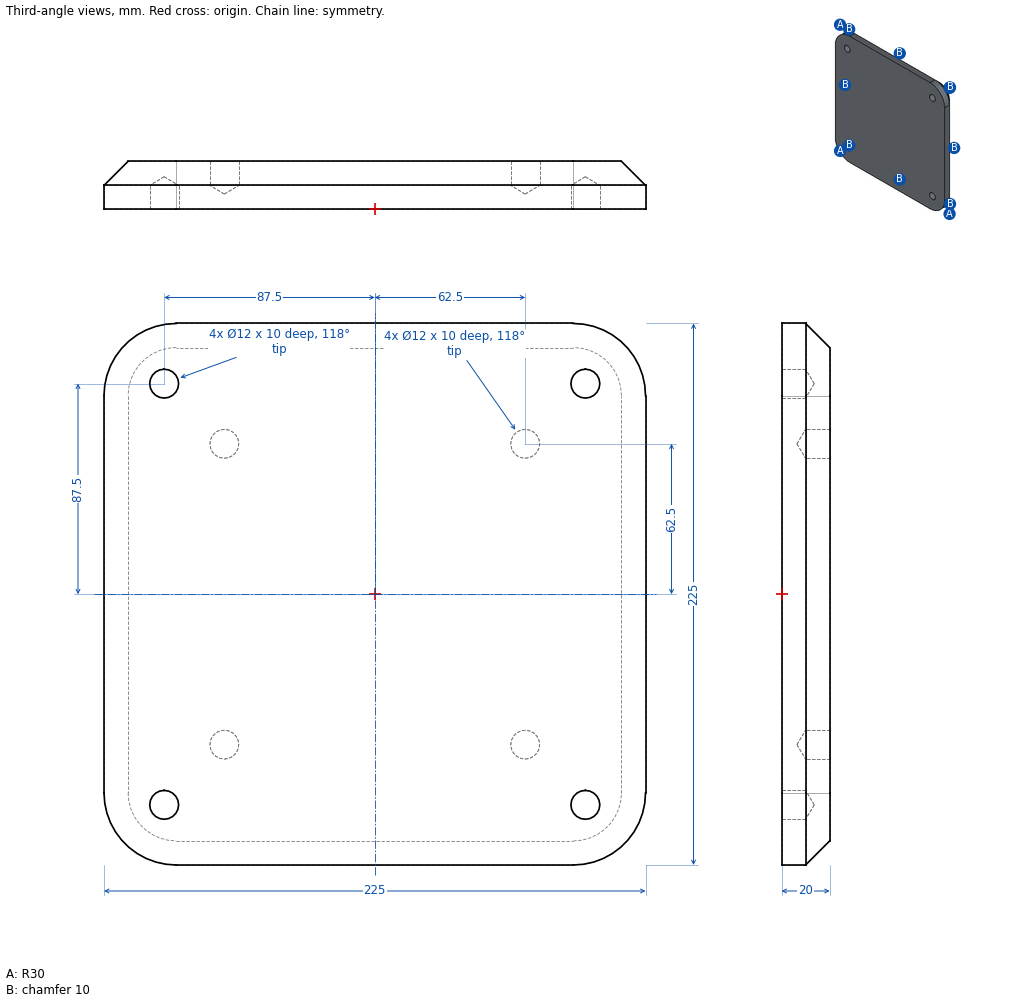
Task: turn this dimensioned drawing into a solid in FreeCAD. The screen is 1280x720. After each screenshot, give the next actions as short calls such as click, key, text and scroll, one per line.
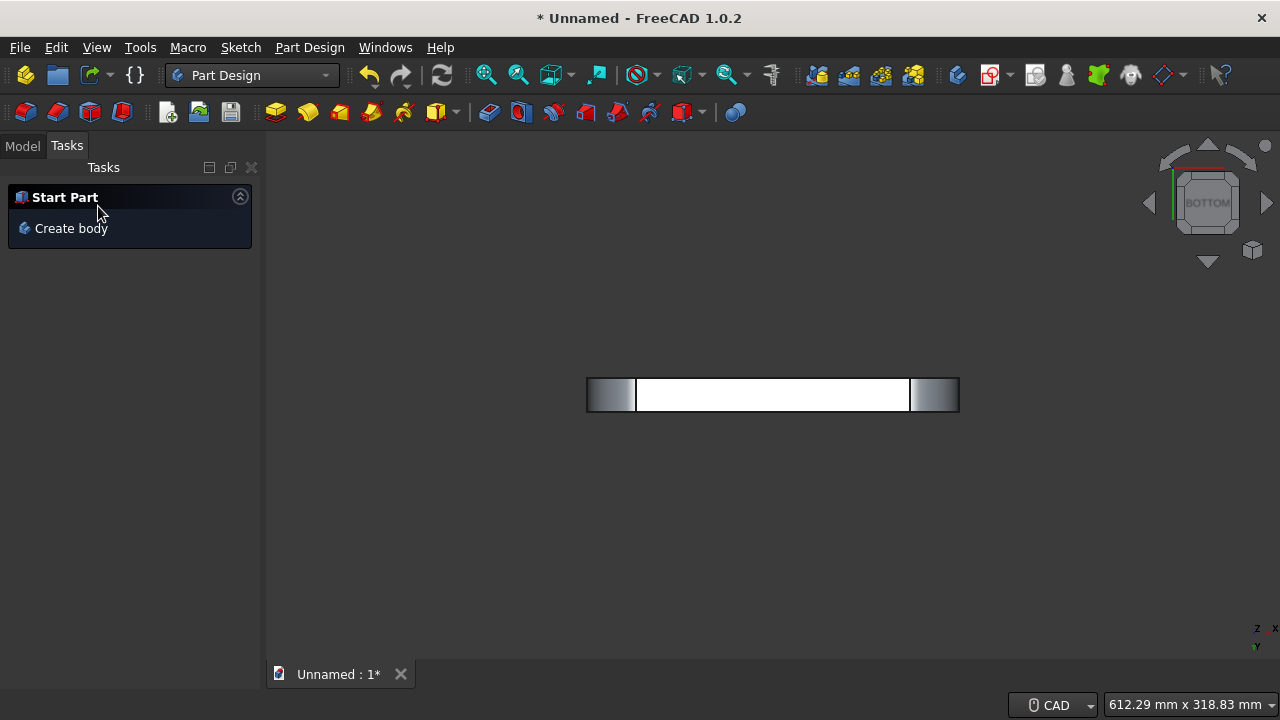
click(488, 76)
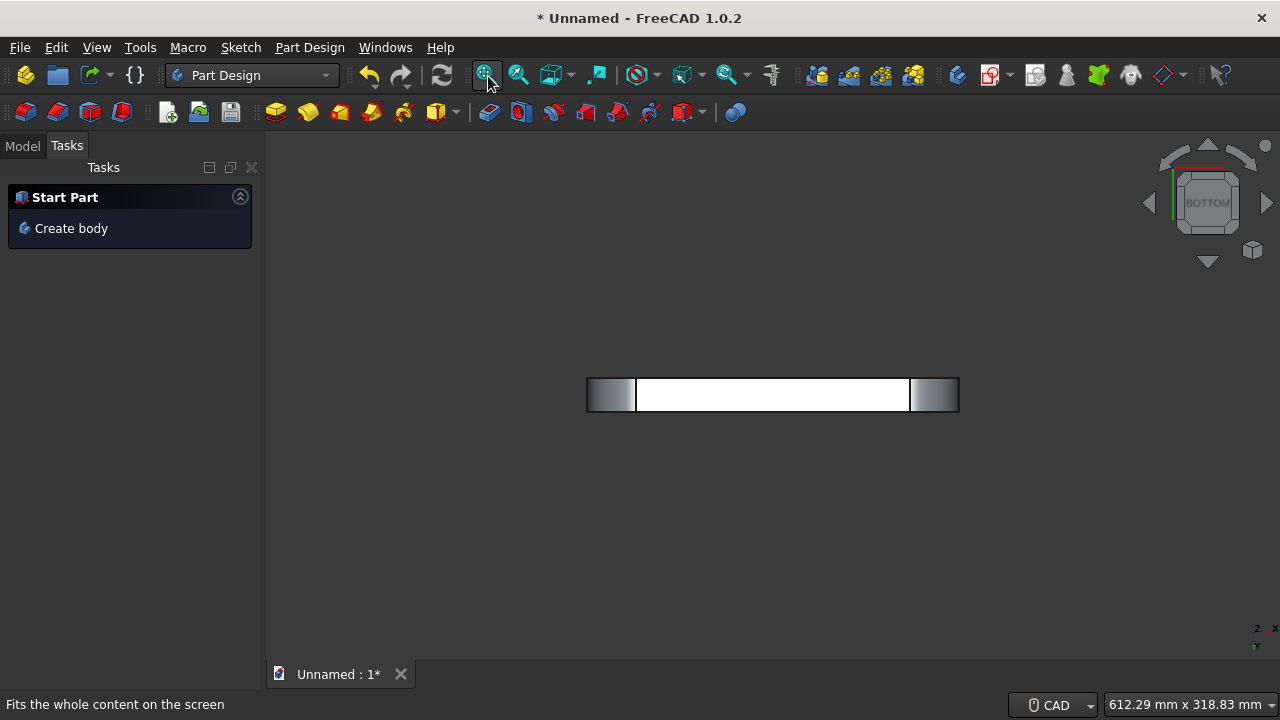
key(0)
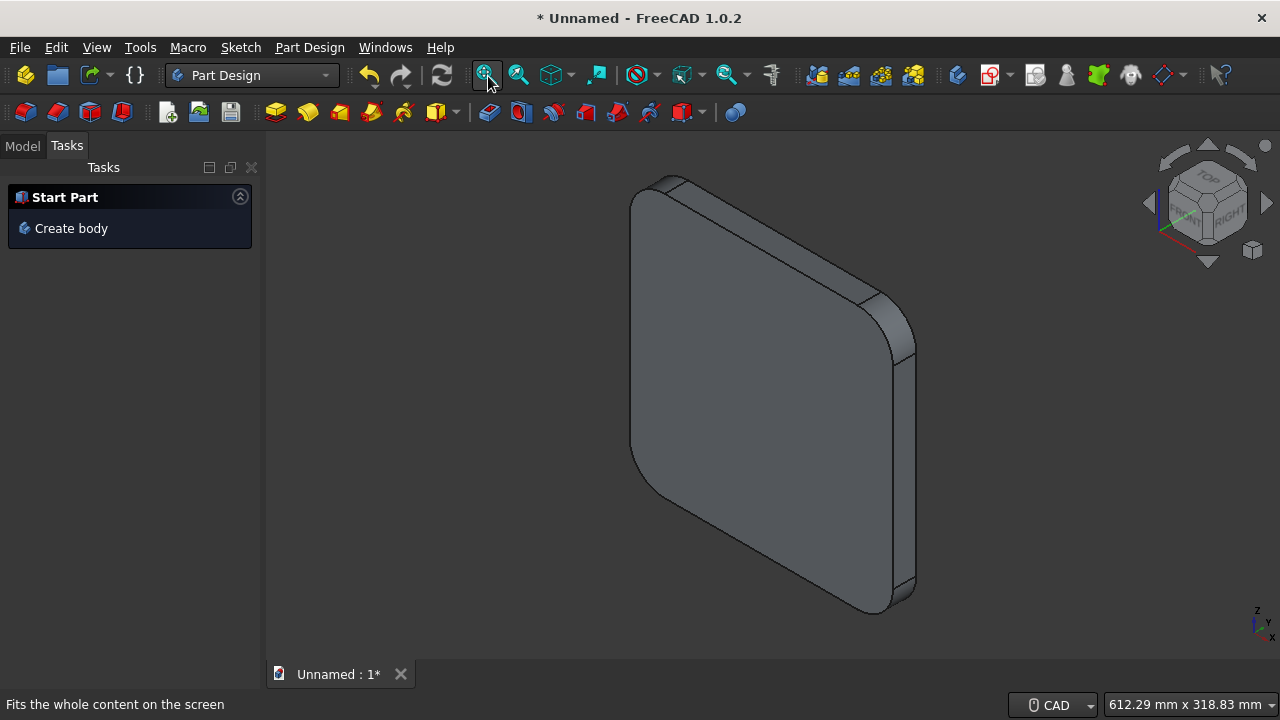
key(2)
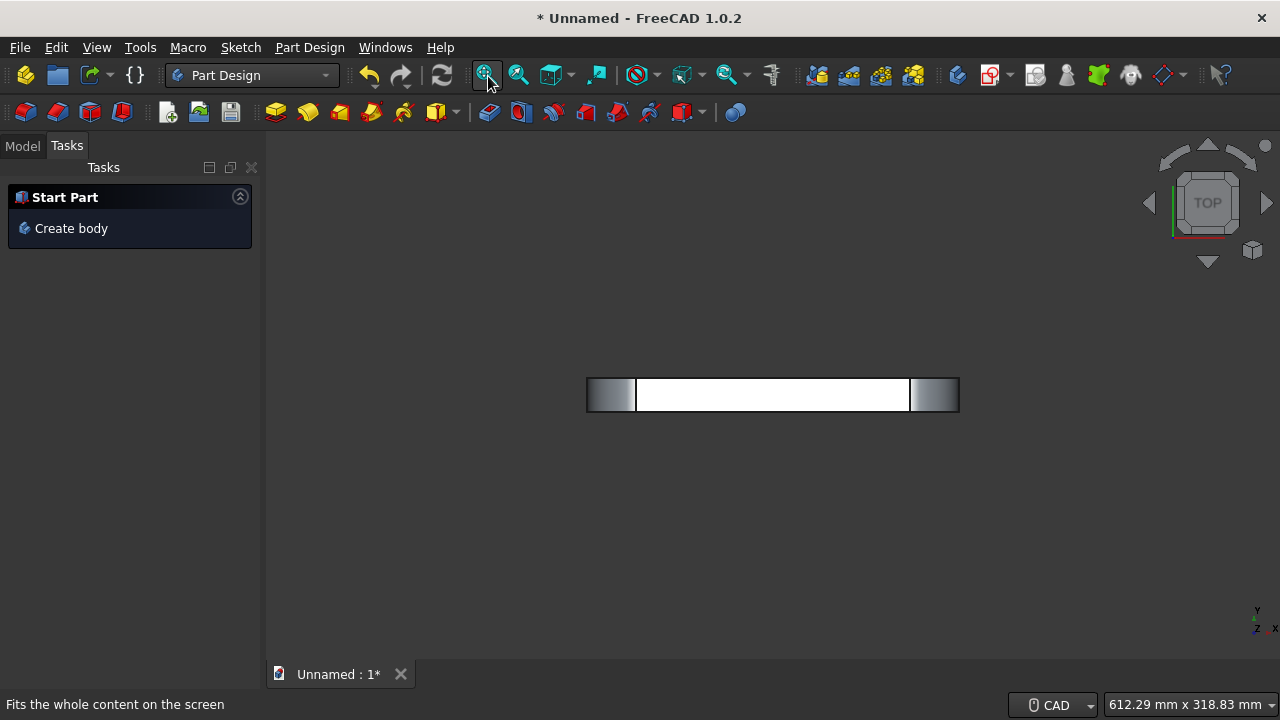
click(488, 76)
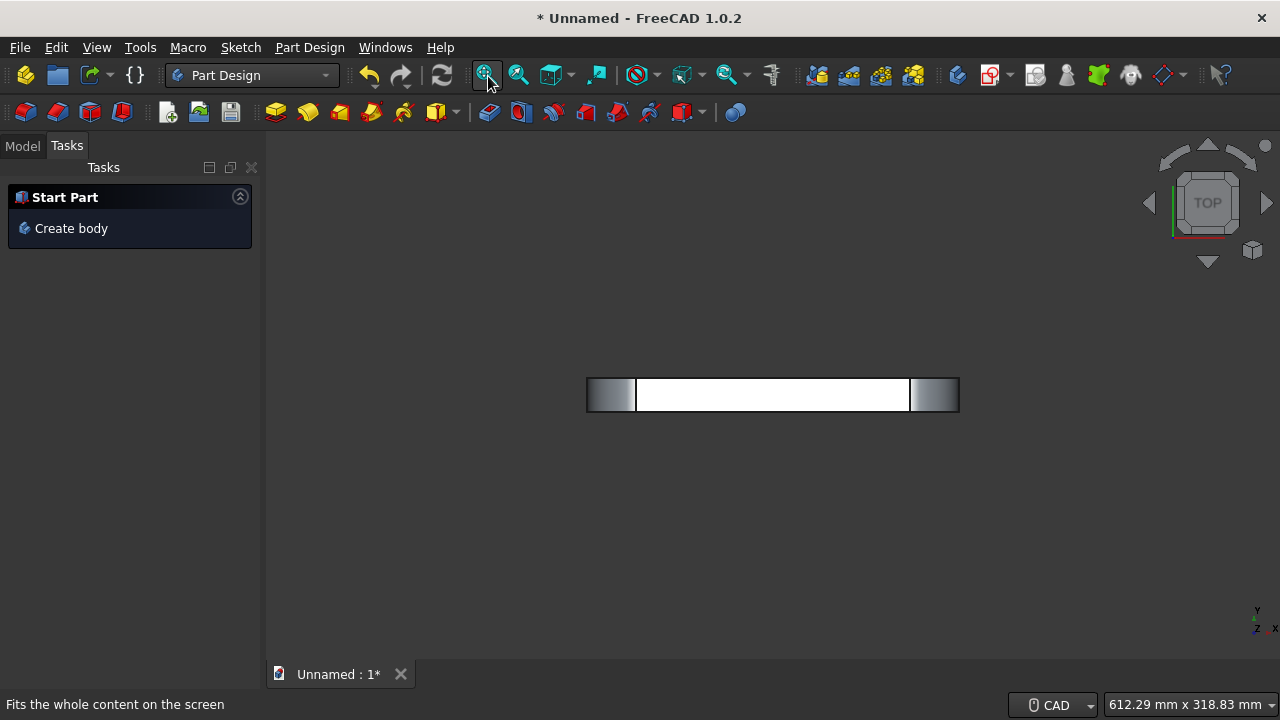
key(1)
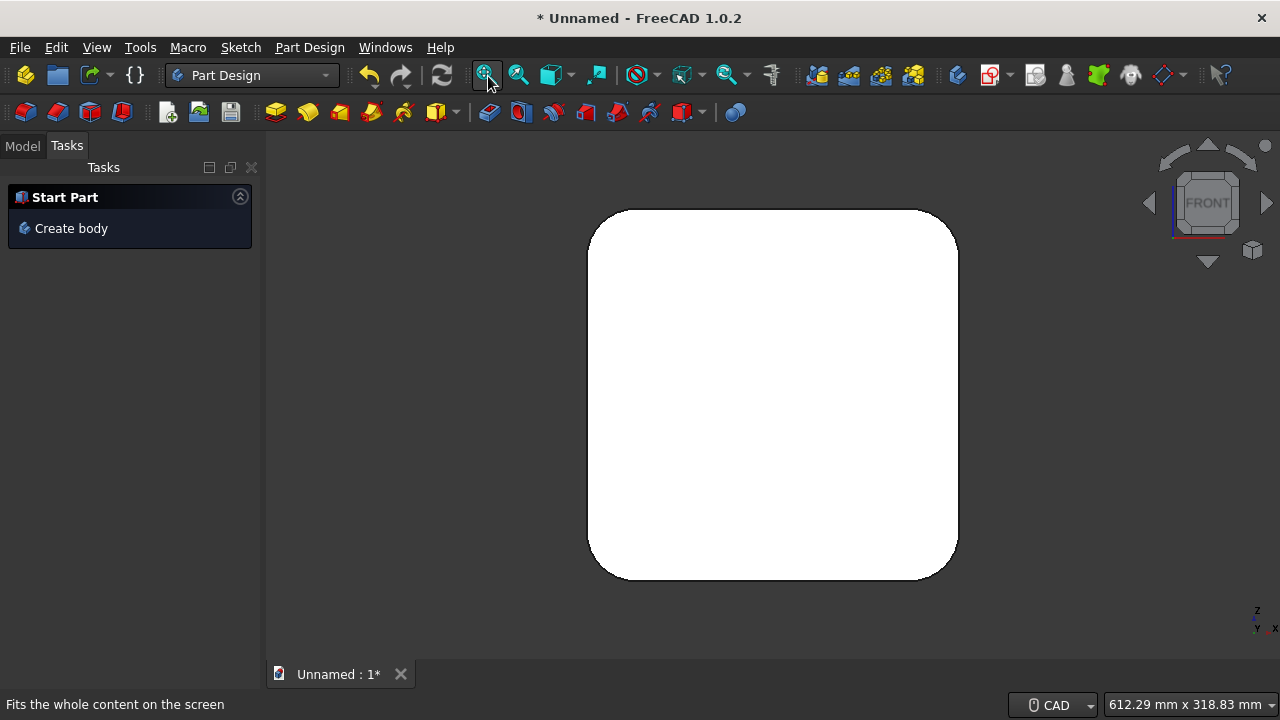
key(3)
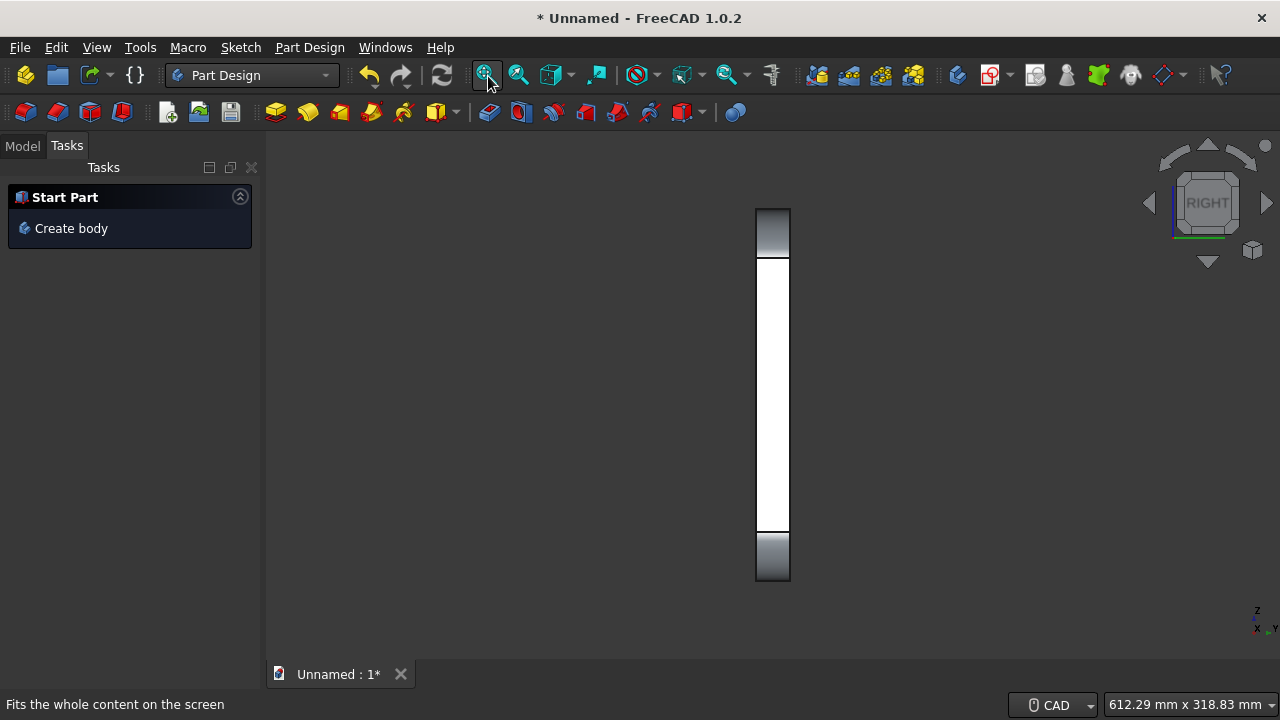
key(5)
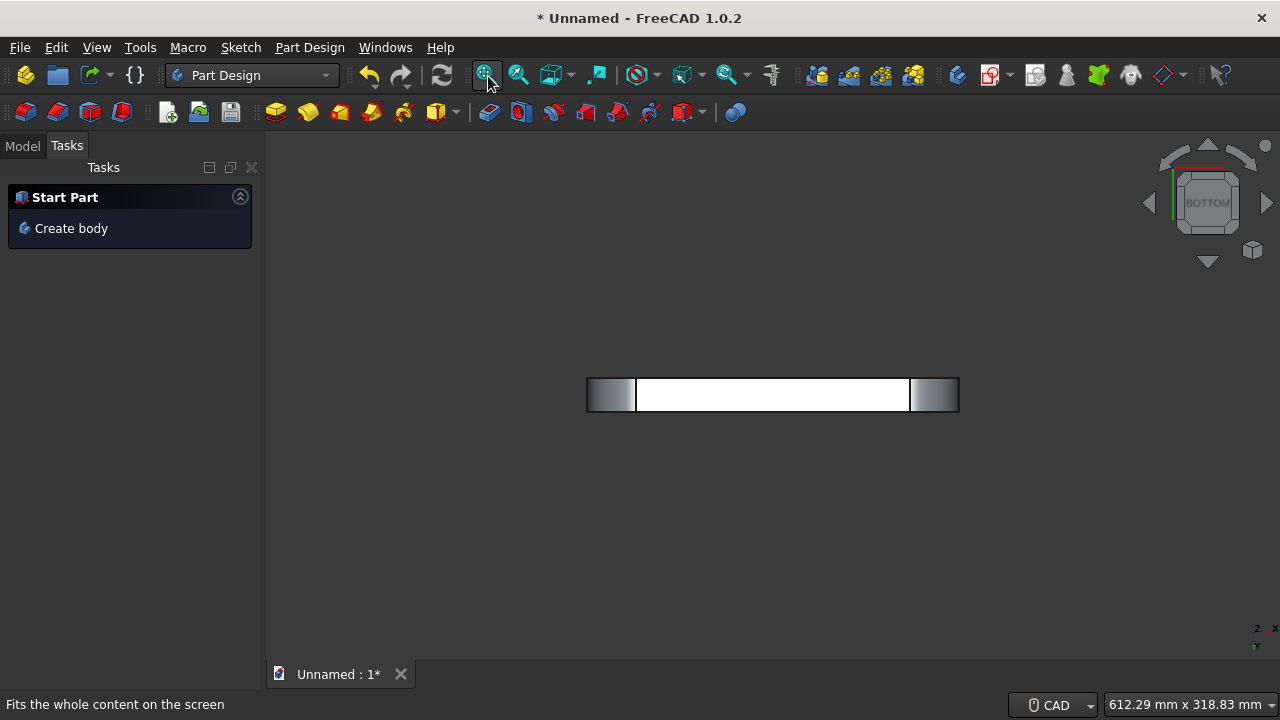
click(488, 76)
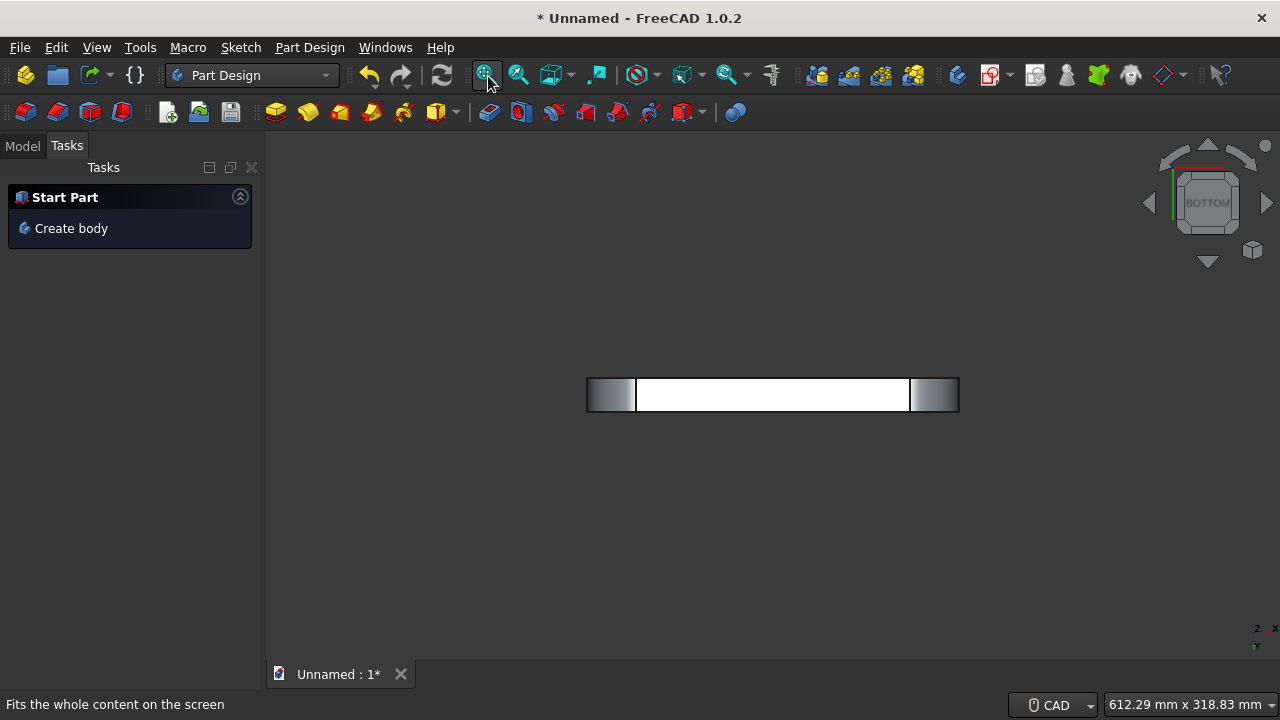
key(4)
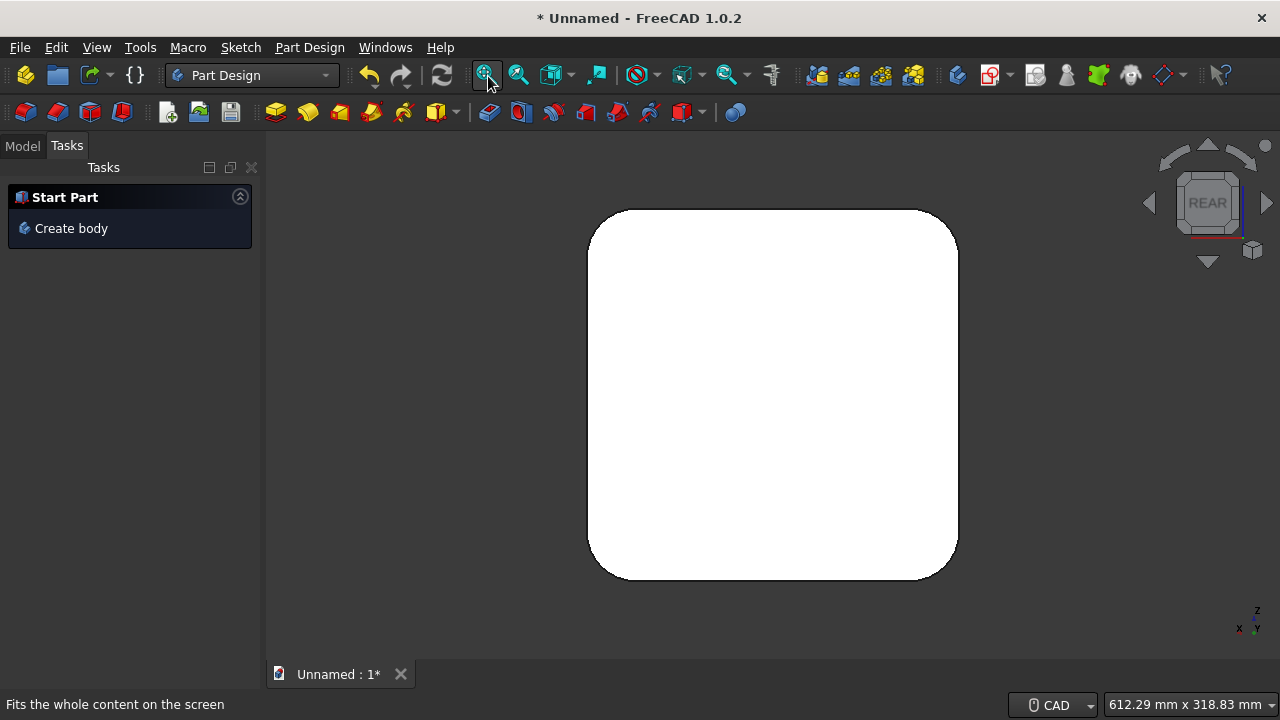
click(773, 394)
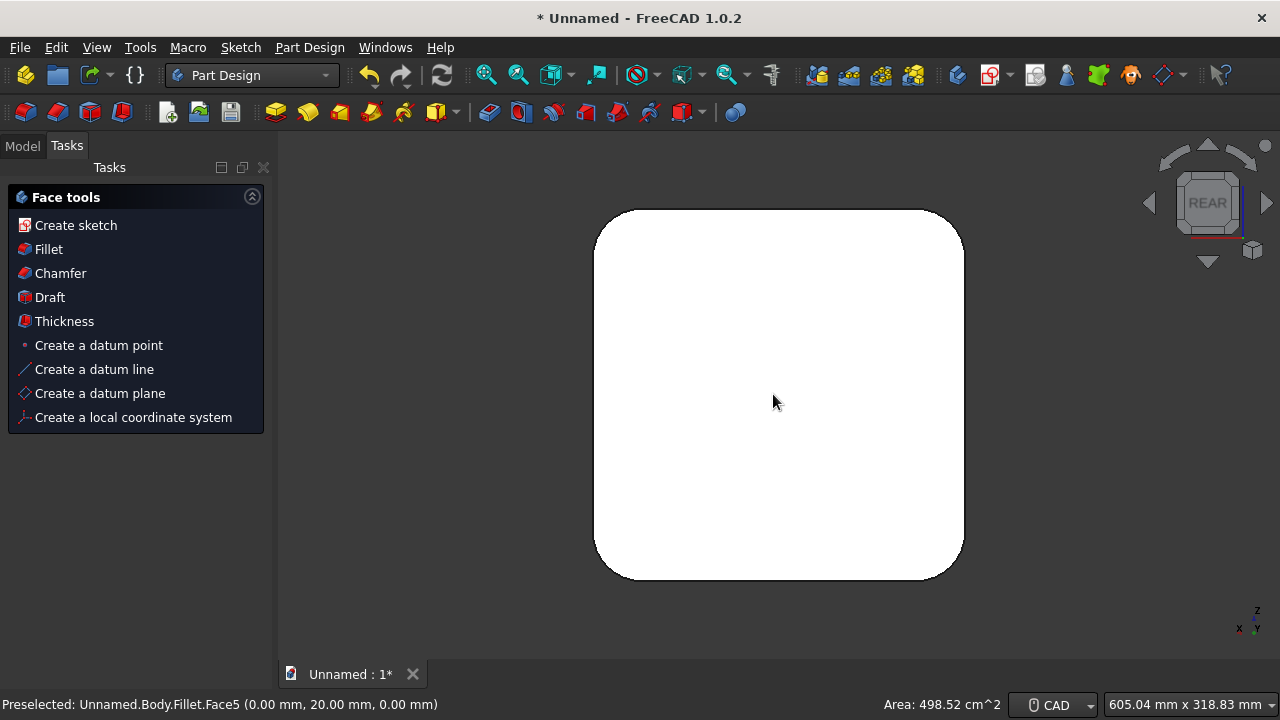
click(58, 112)